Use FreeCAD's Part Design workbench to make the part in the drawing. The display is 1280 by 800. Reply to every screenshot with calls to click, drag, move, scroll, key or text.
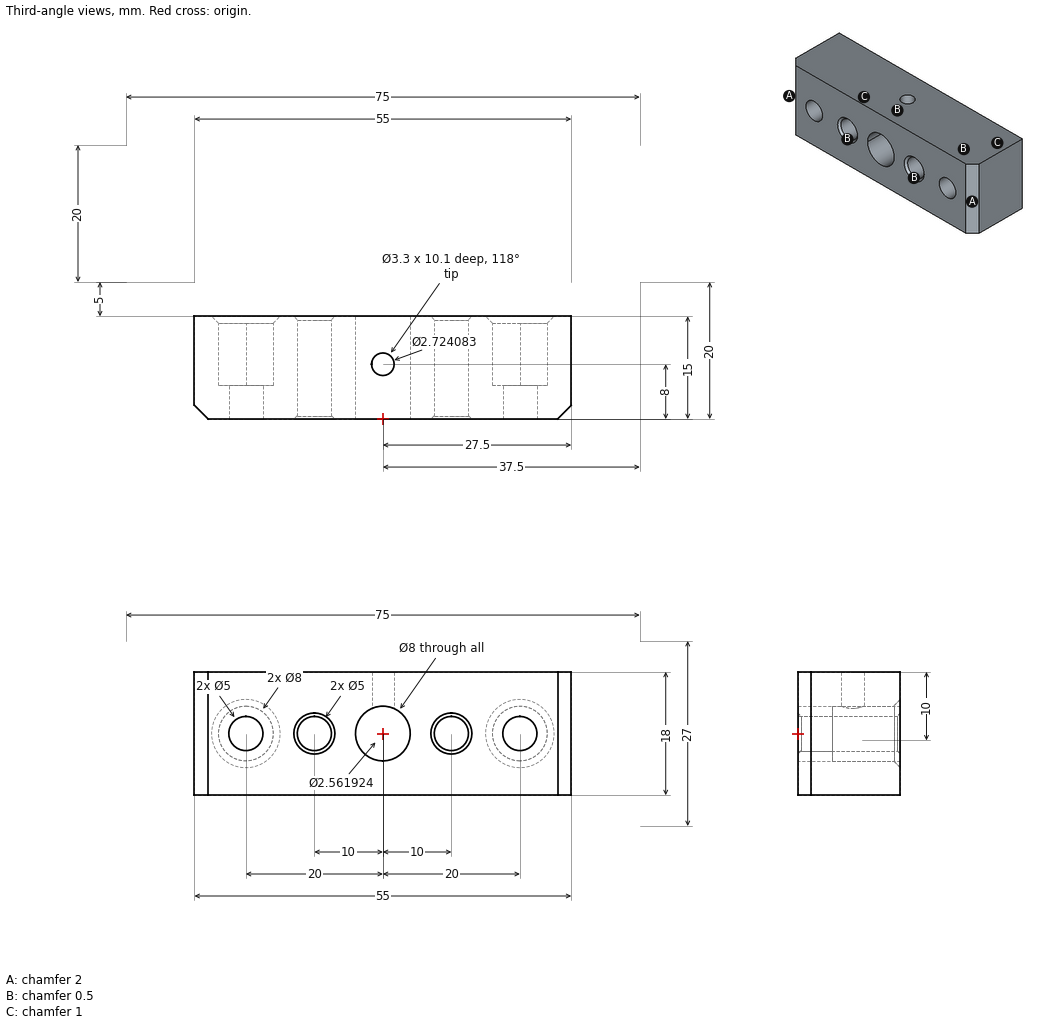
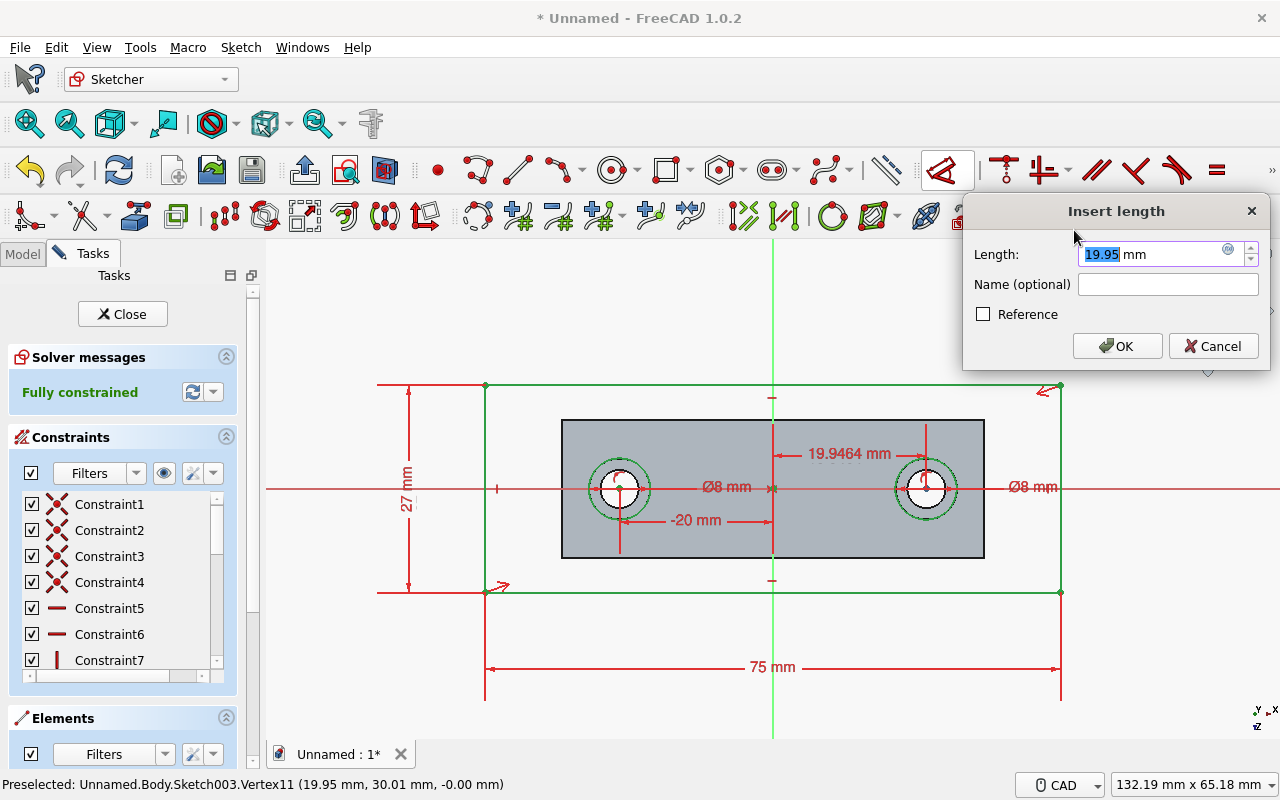
text(20)
key(Return)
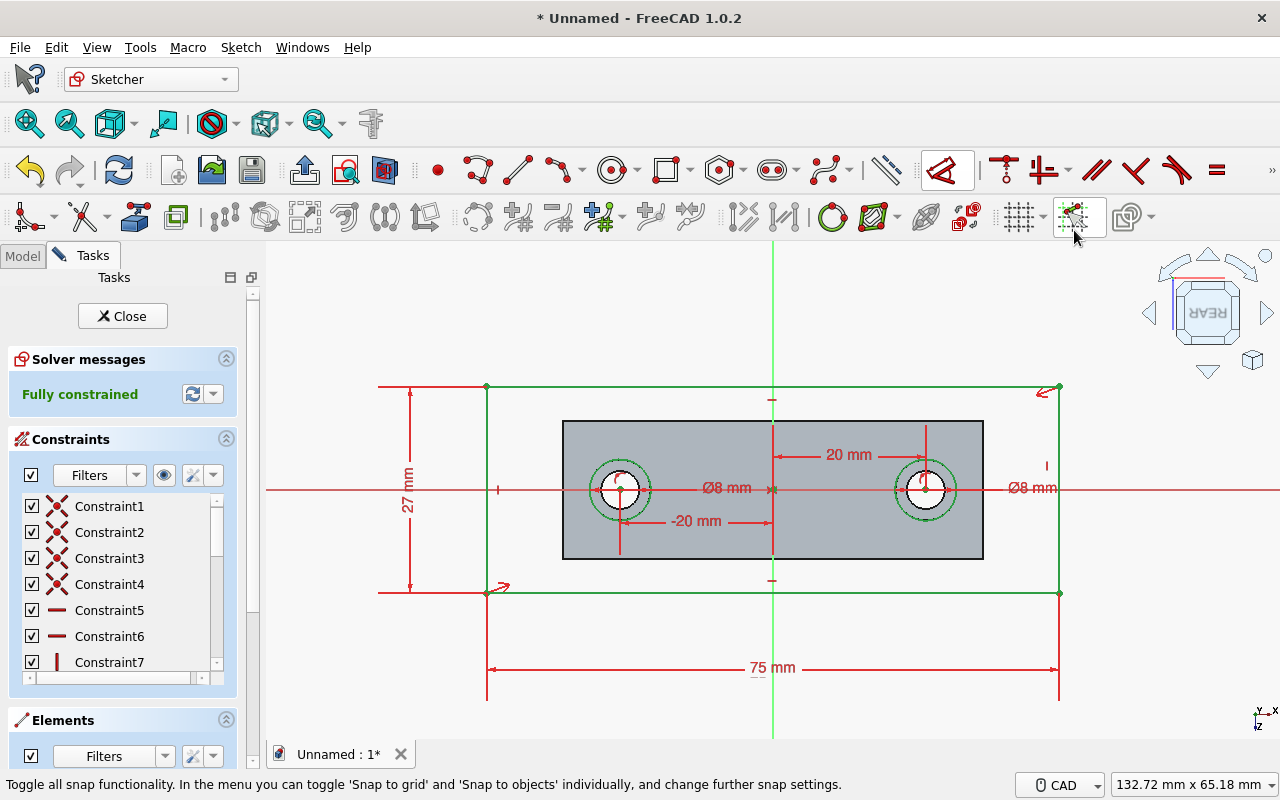
click(123, 316)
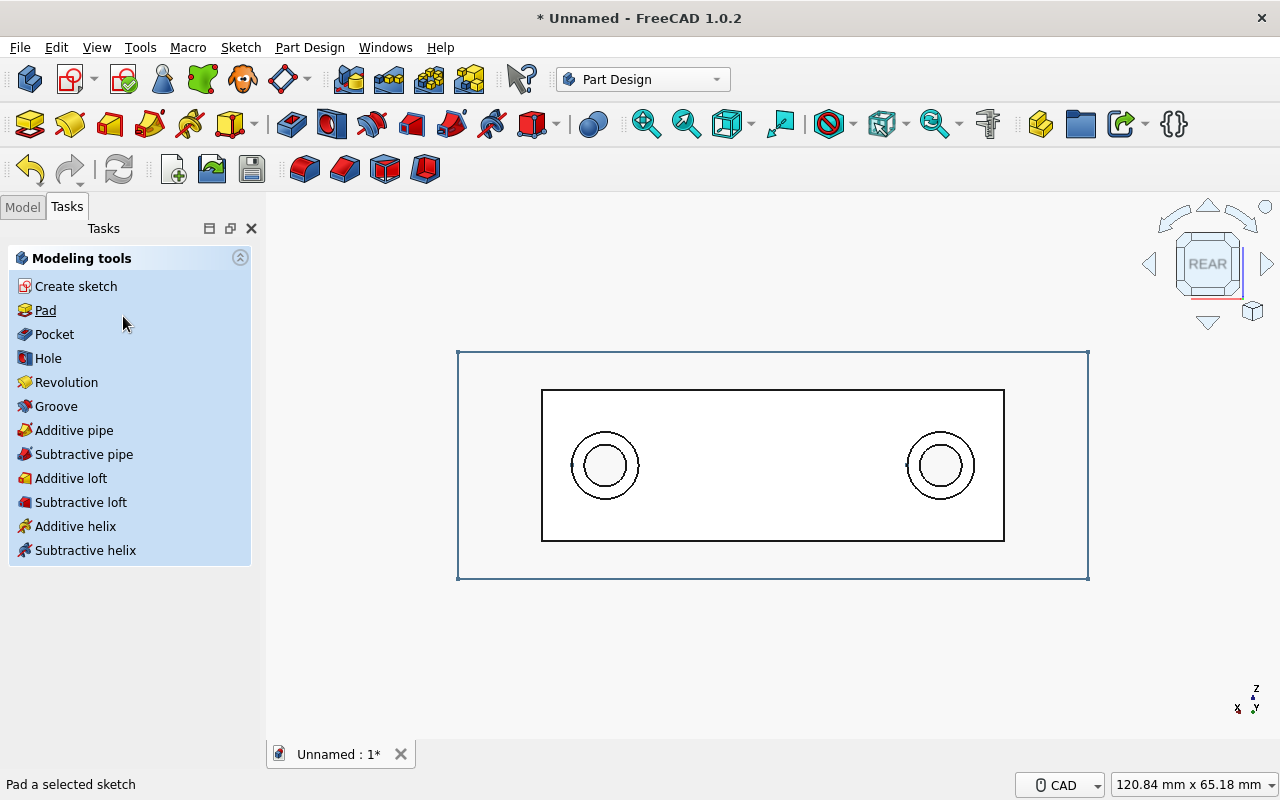
click(30, 124)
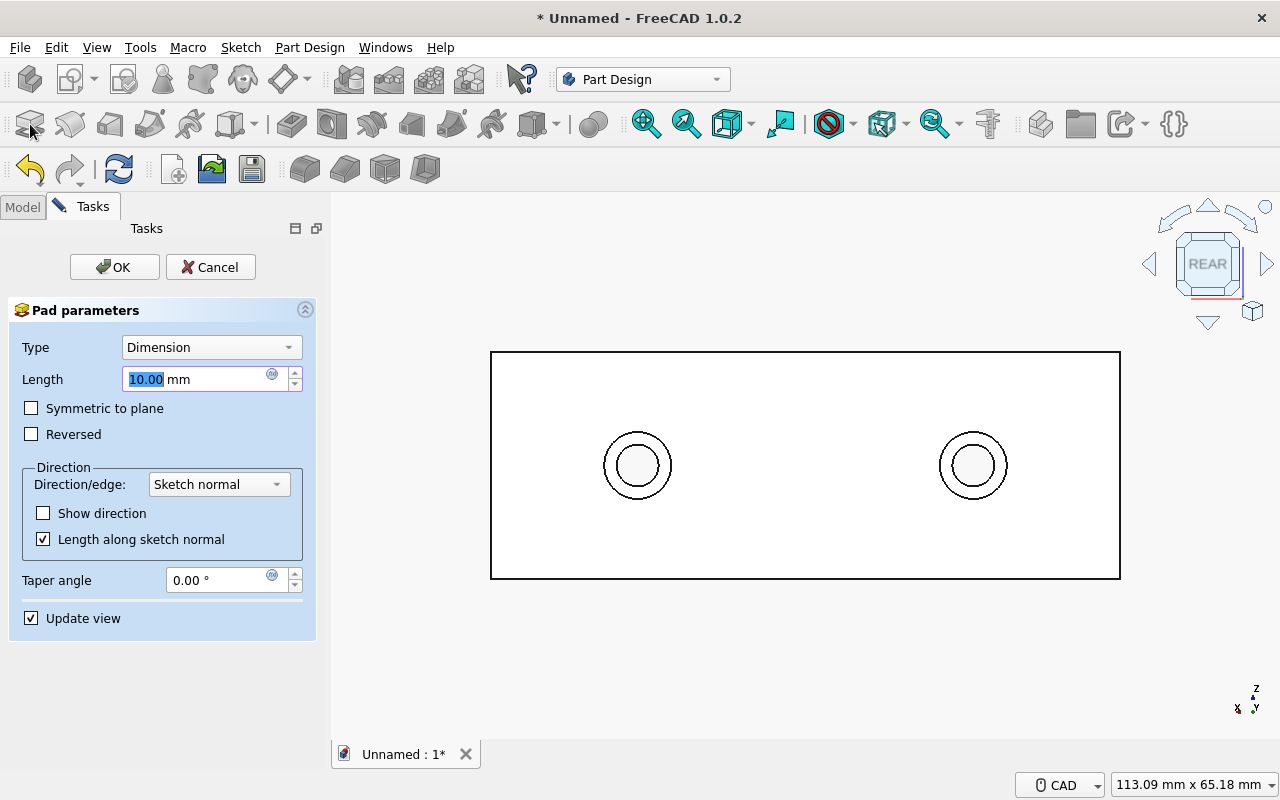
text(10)
key(Tab)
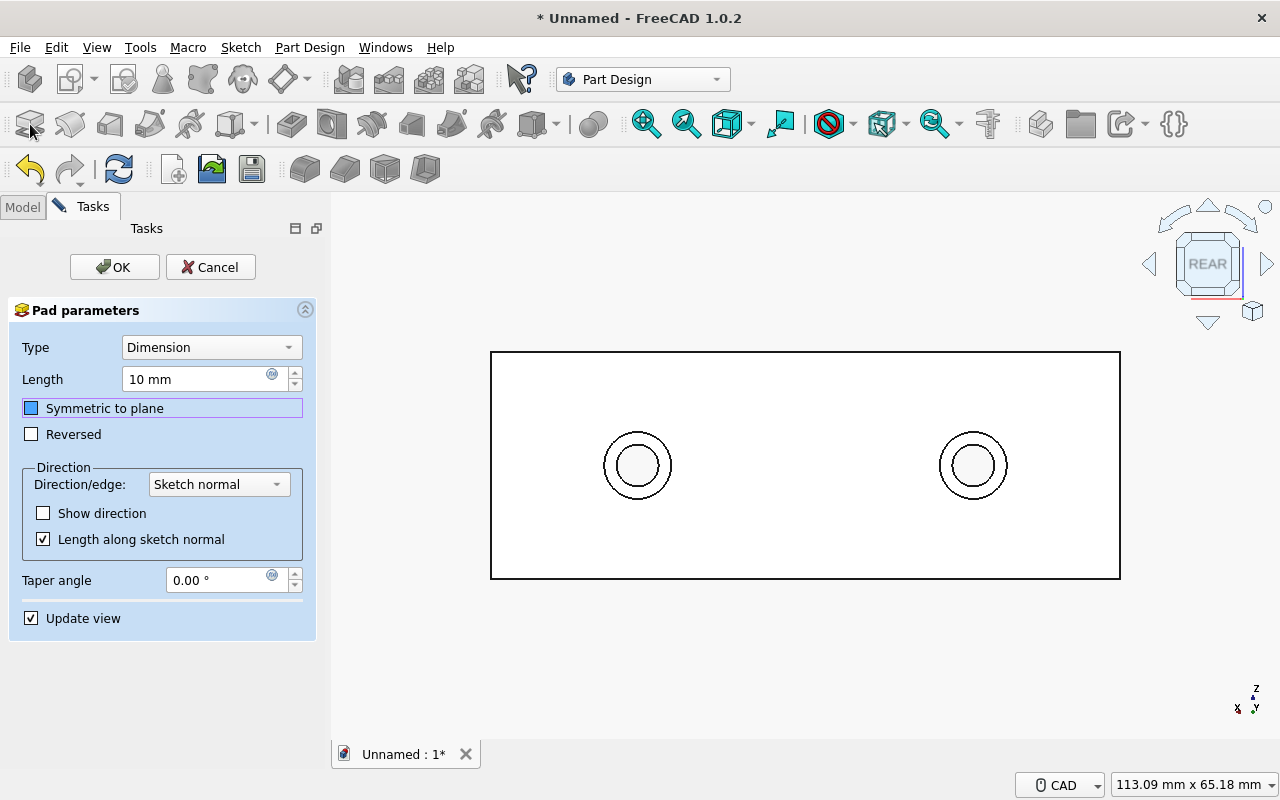
click(30, 434)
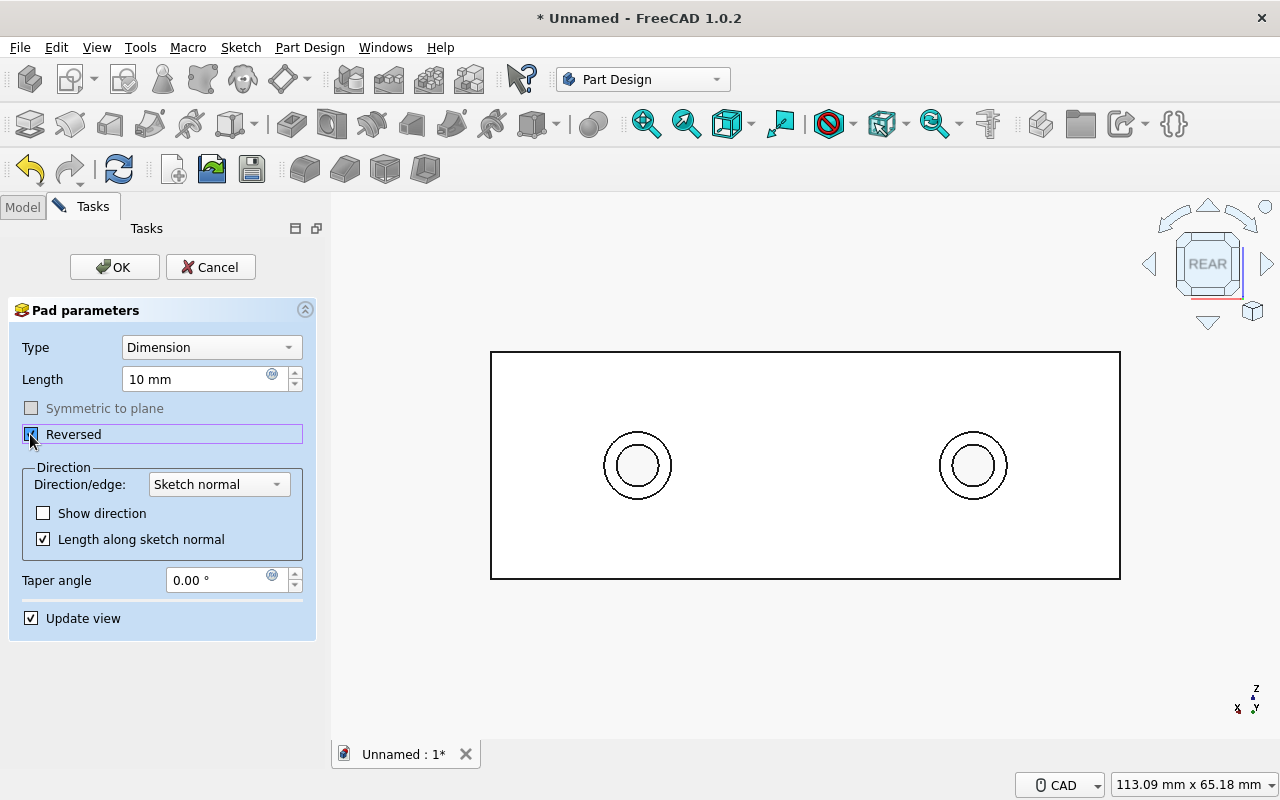
click(115, 267)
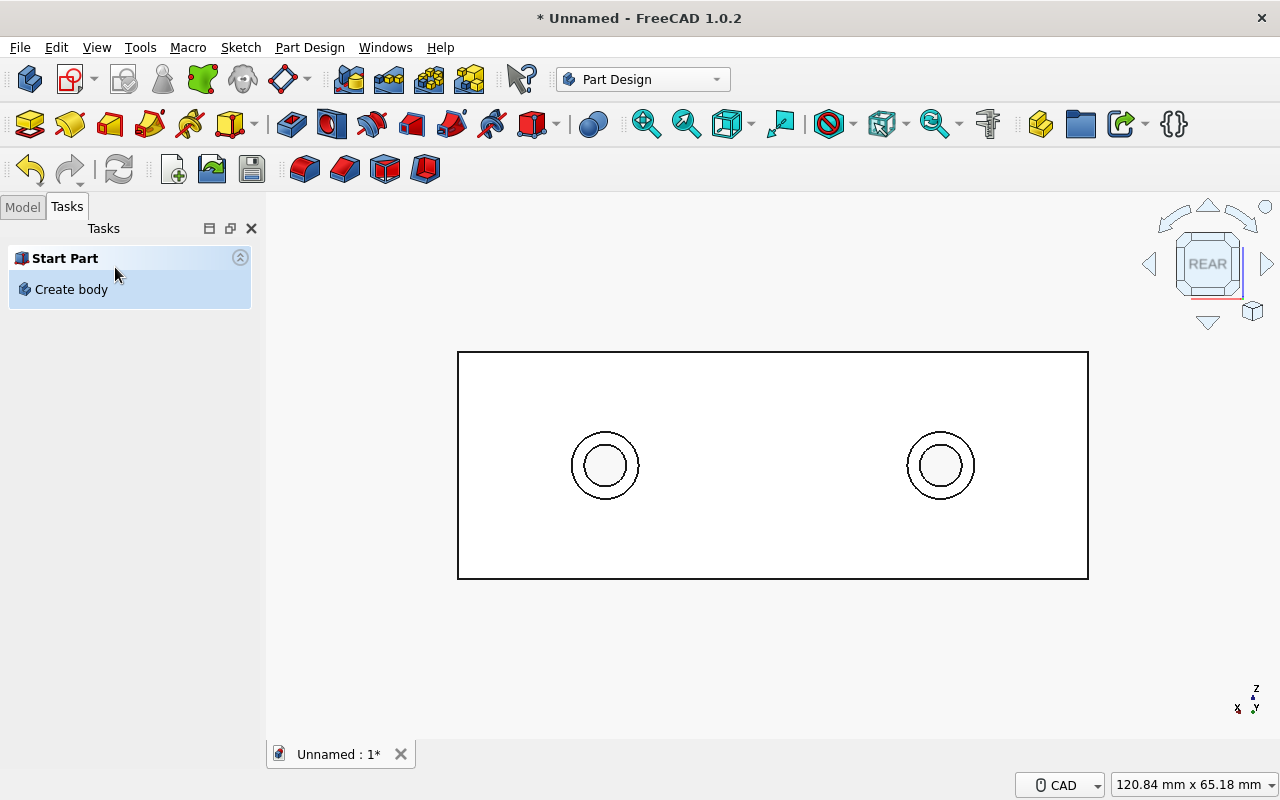
click(23, 206)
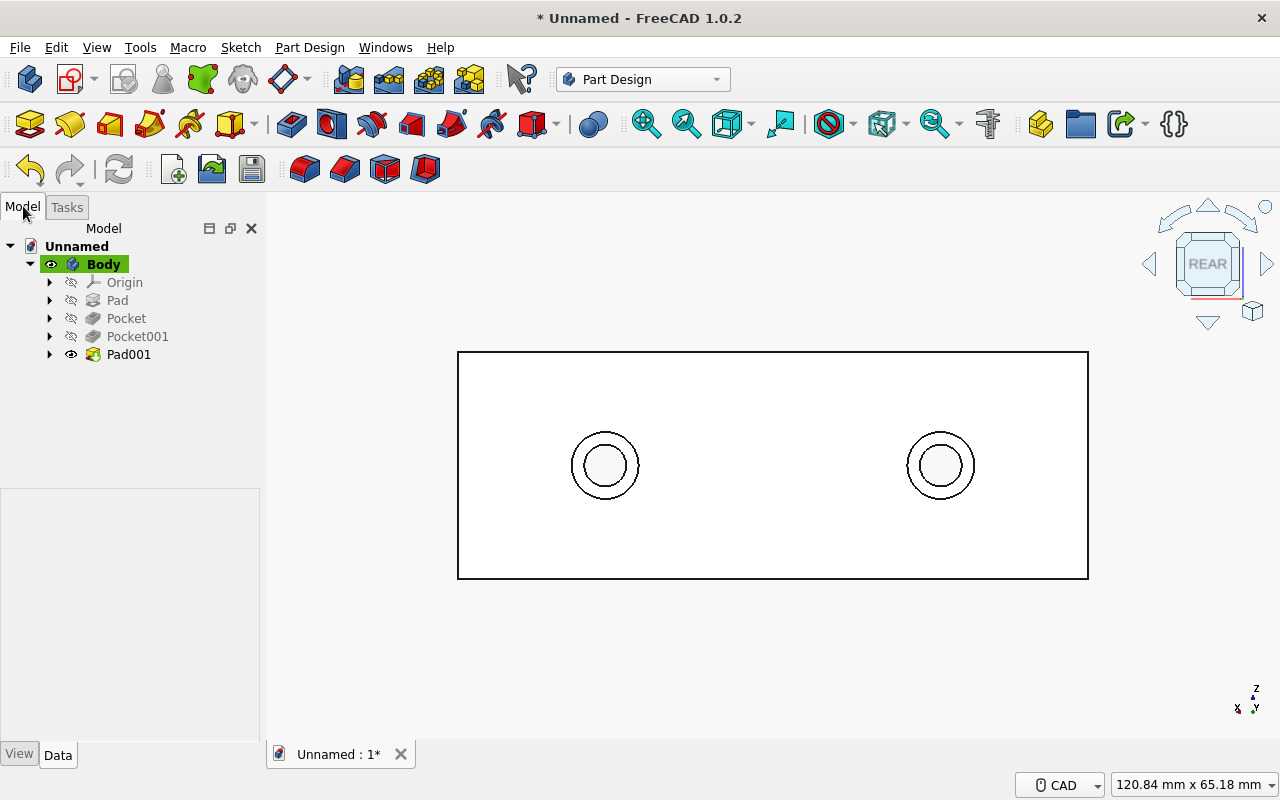
click(50, 282)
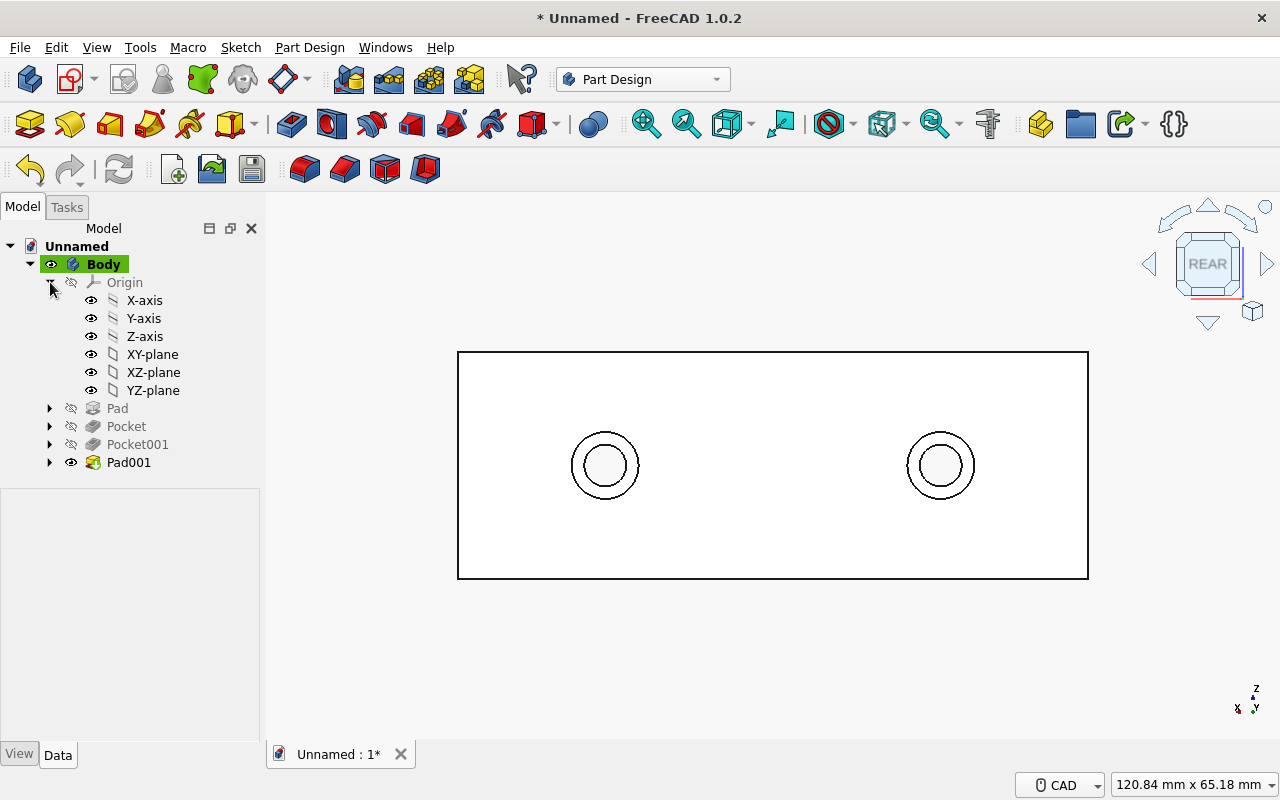
click(136, 372)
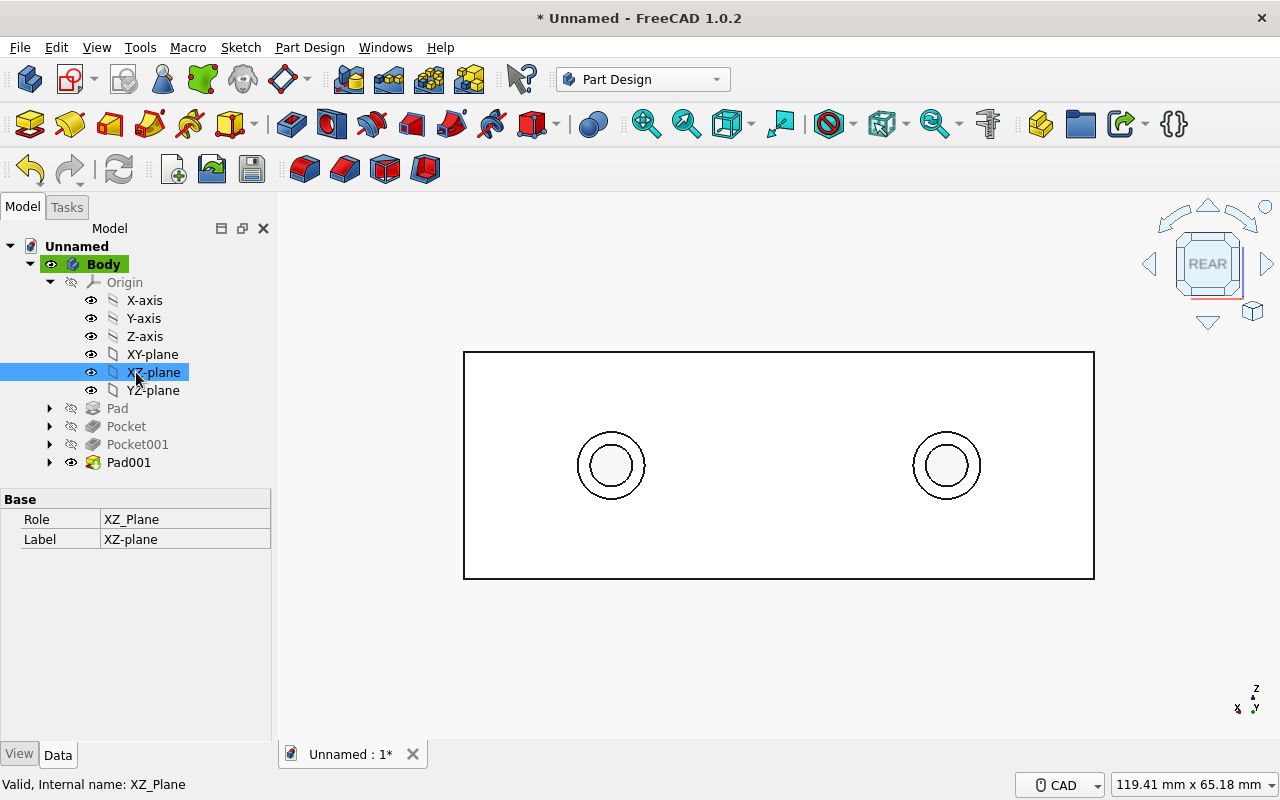
click(284, 80)